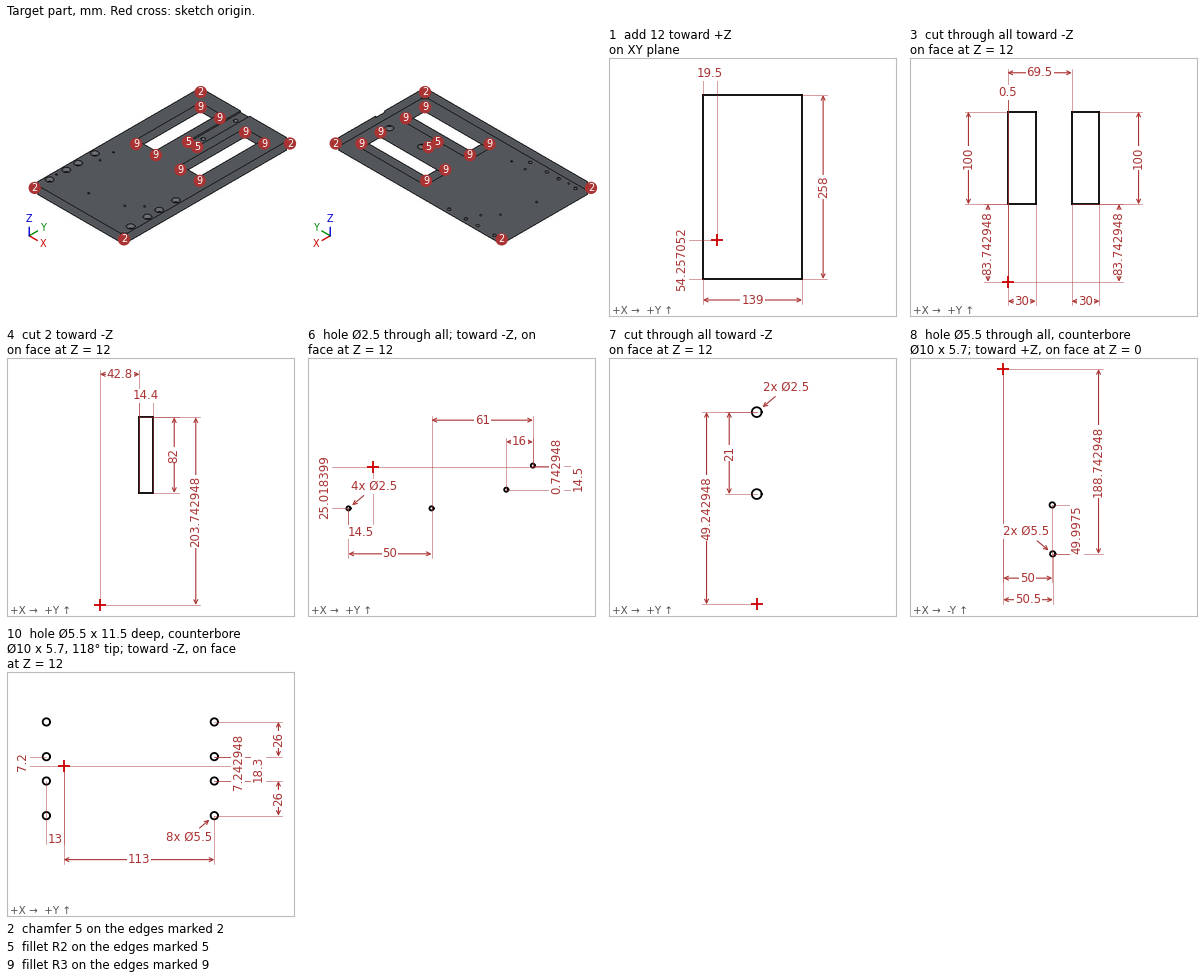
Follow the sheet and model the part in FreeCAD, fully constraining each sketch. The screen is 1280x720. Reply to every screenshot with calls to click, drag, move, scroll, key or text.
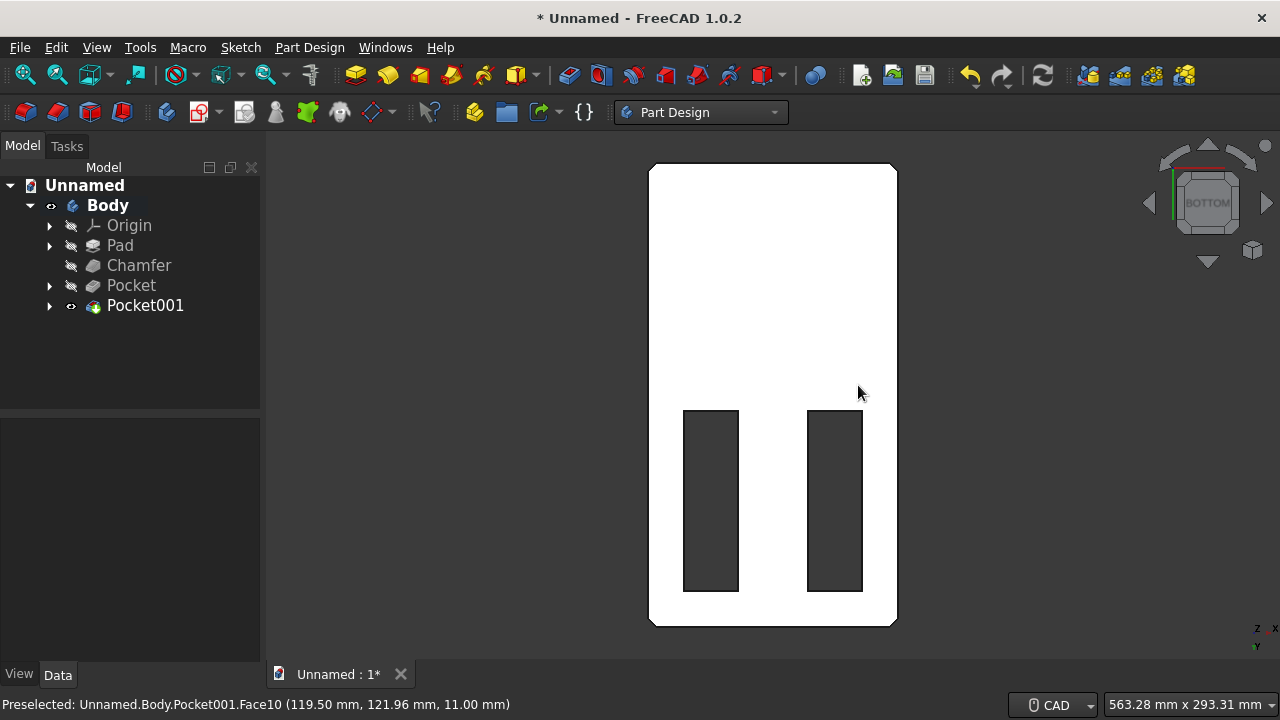
scroll(786, 479, up, 13)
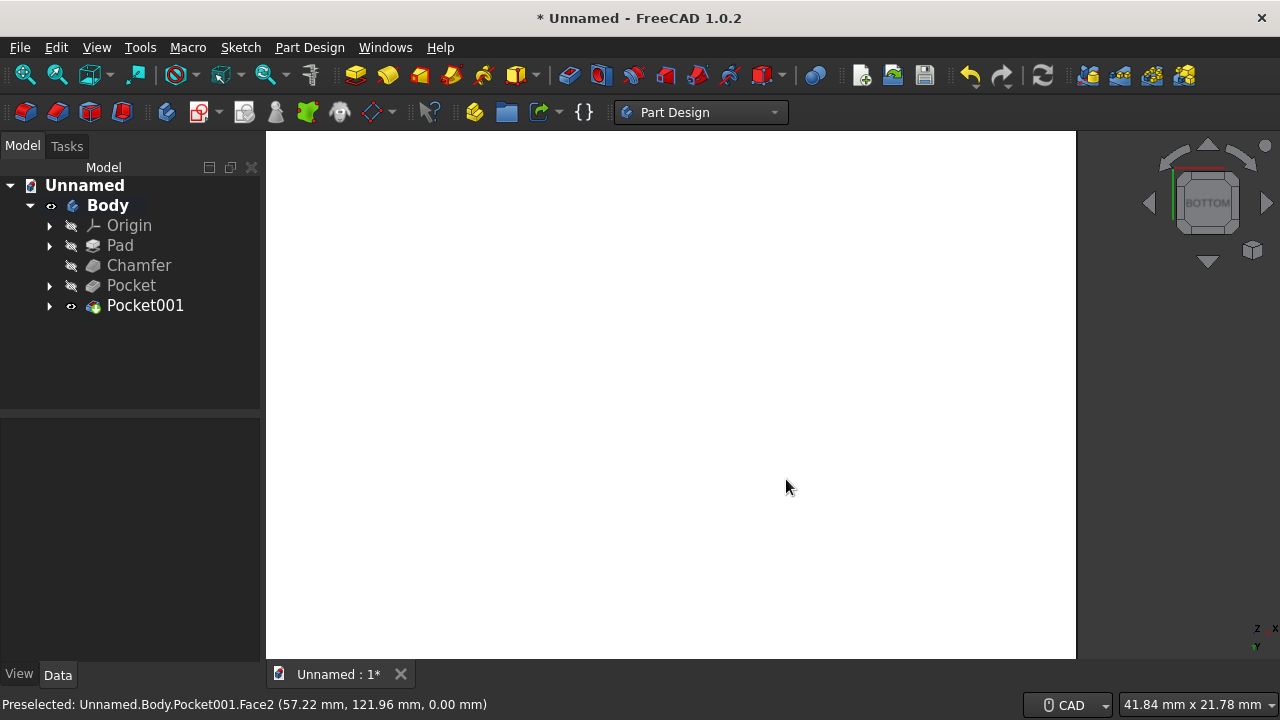
key(v)
key(f)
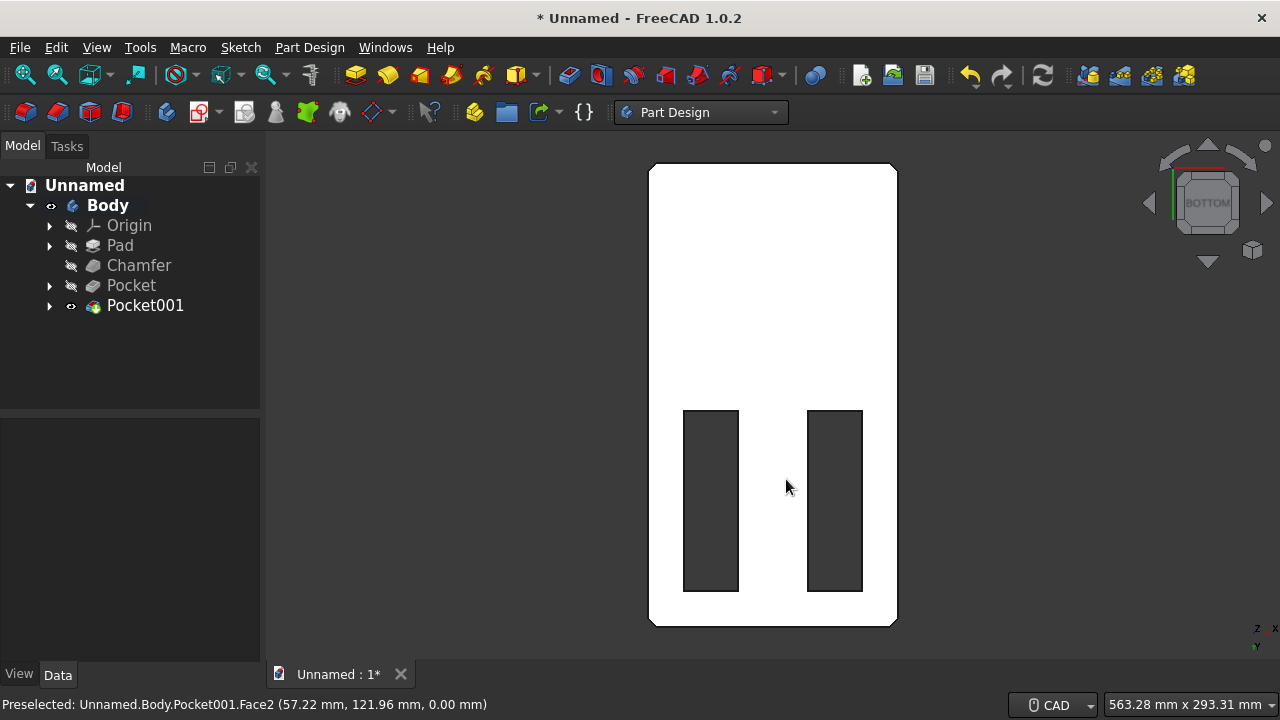
key(4)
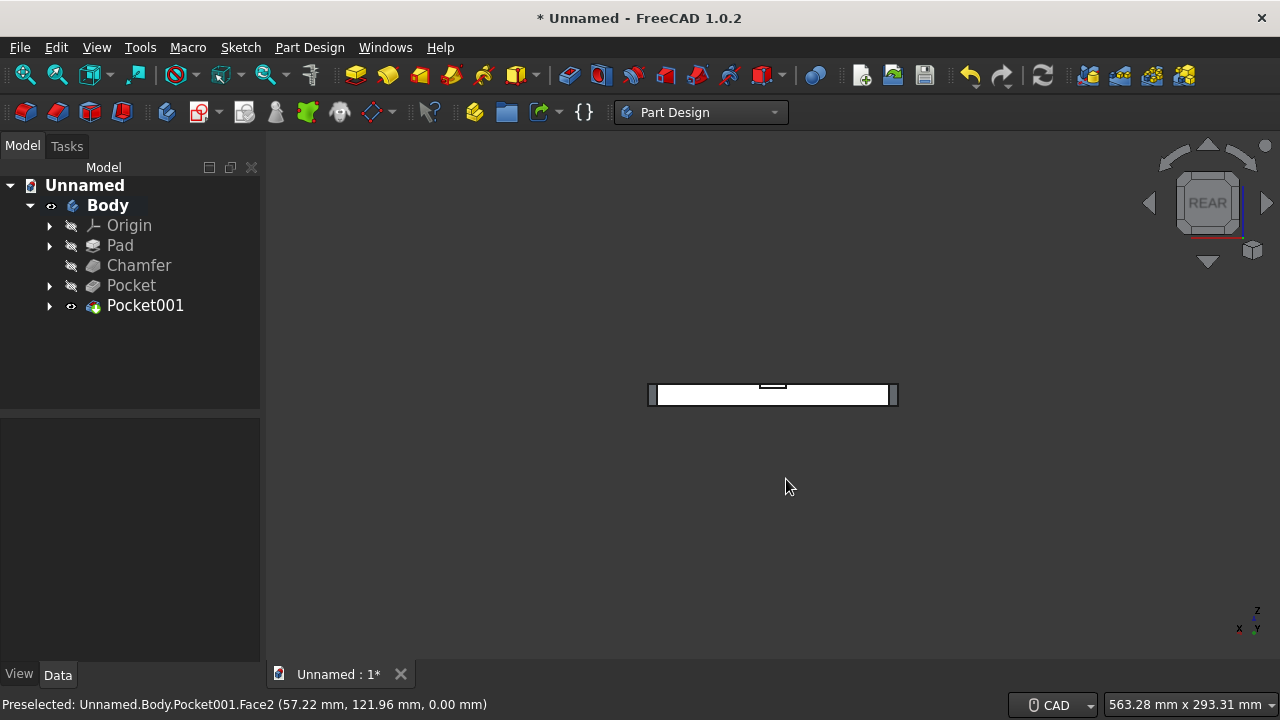
key(v)
key(f)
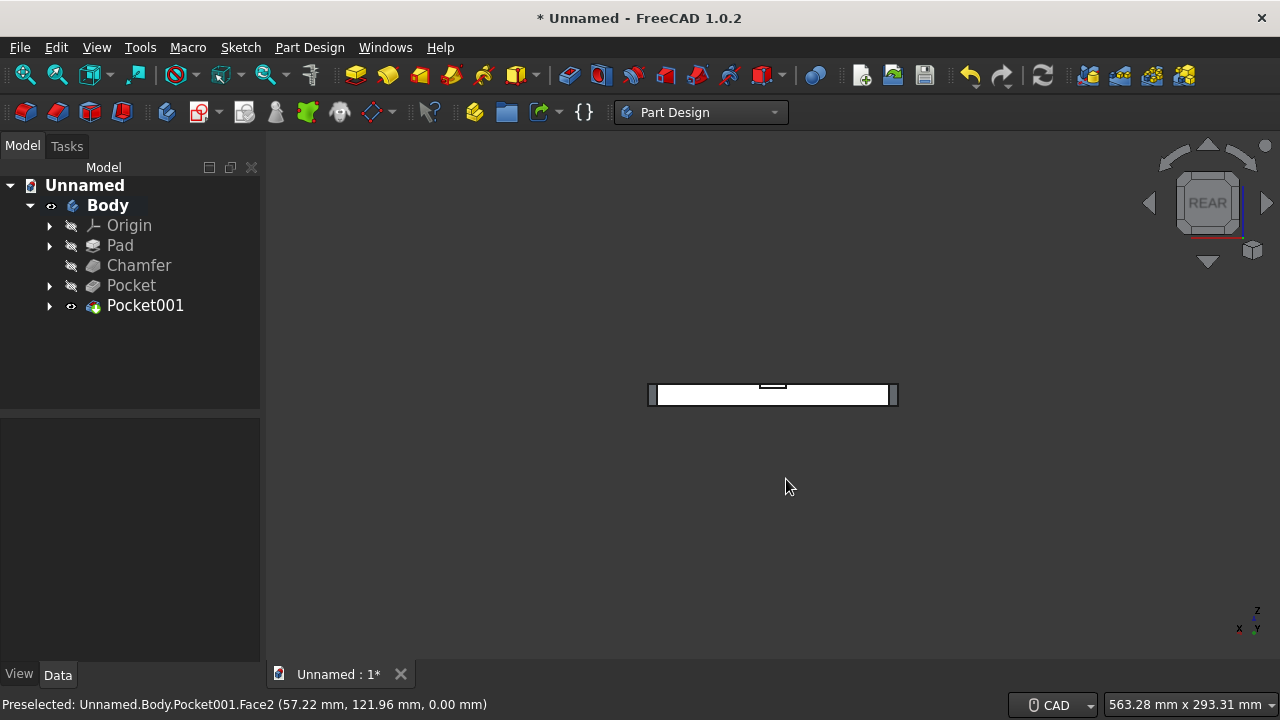
scroll(760, 385, up, 13)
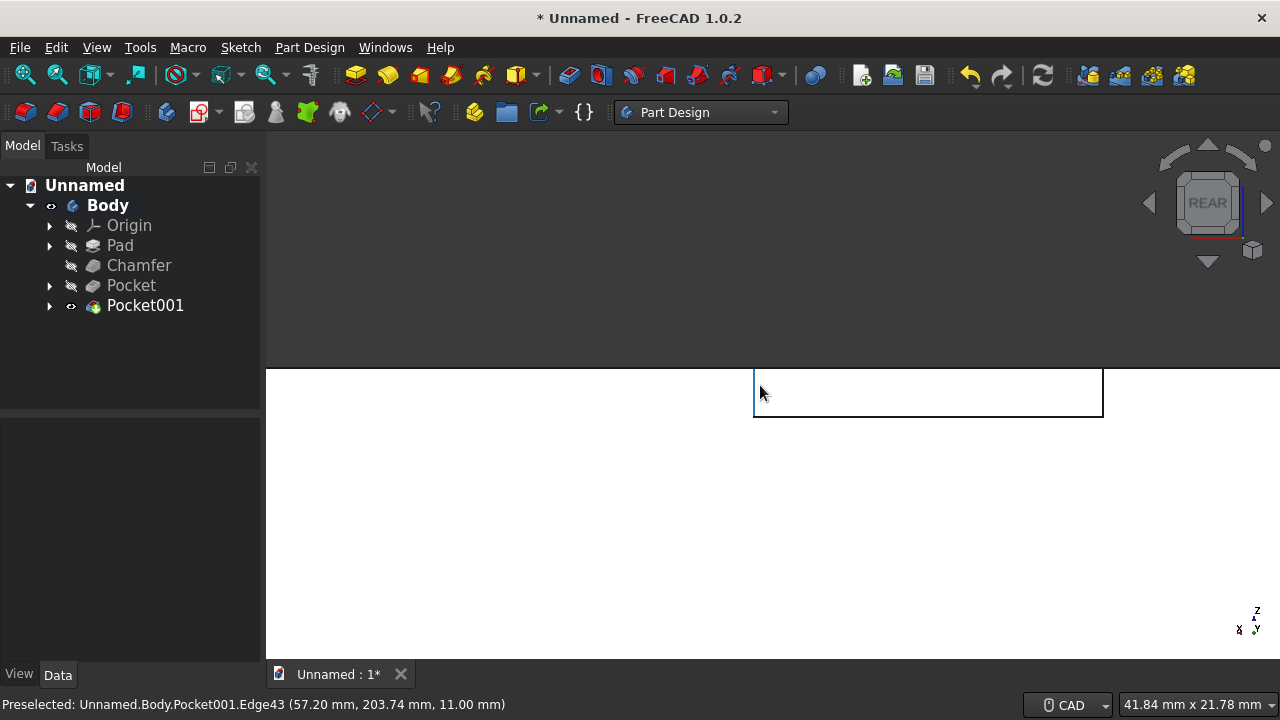
key(v)
key(f)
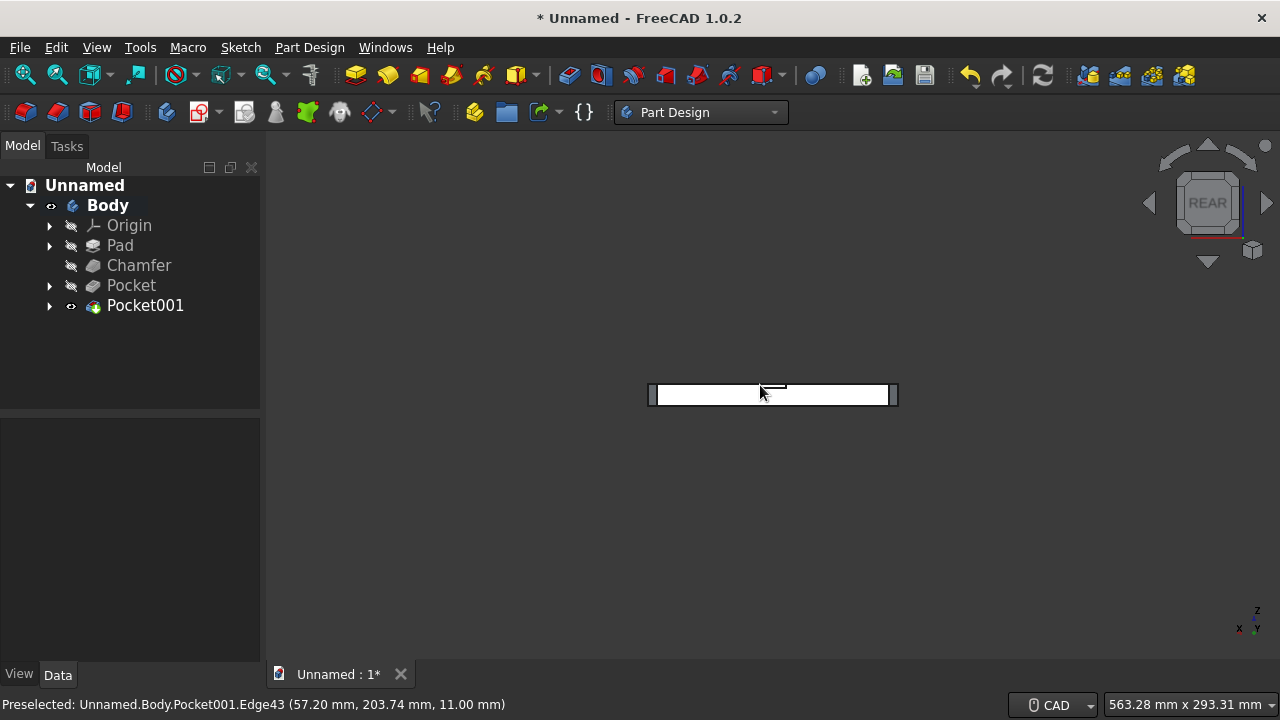
key(6)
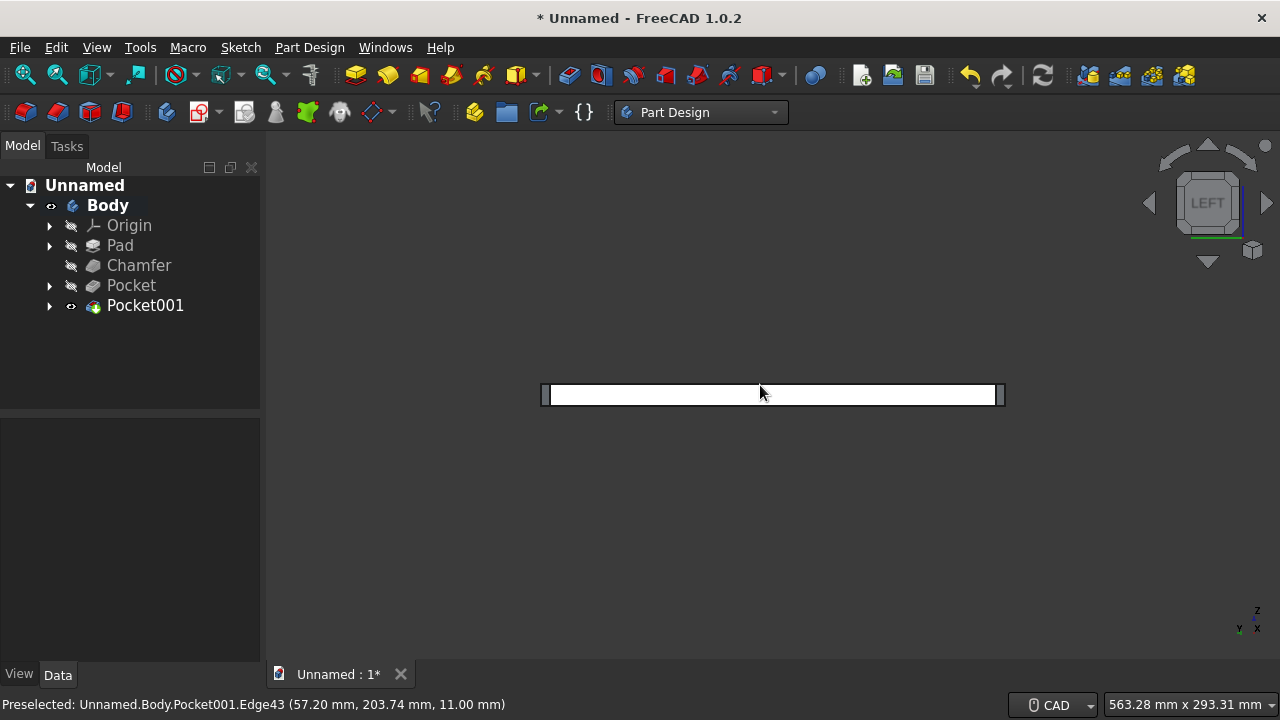
scroll(688, 385, up, 13)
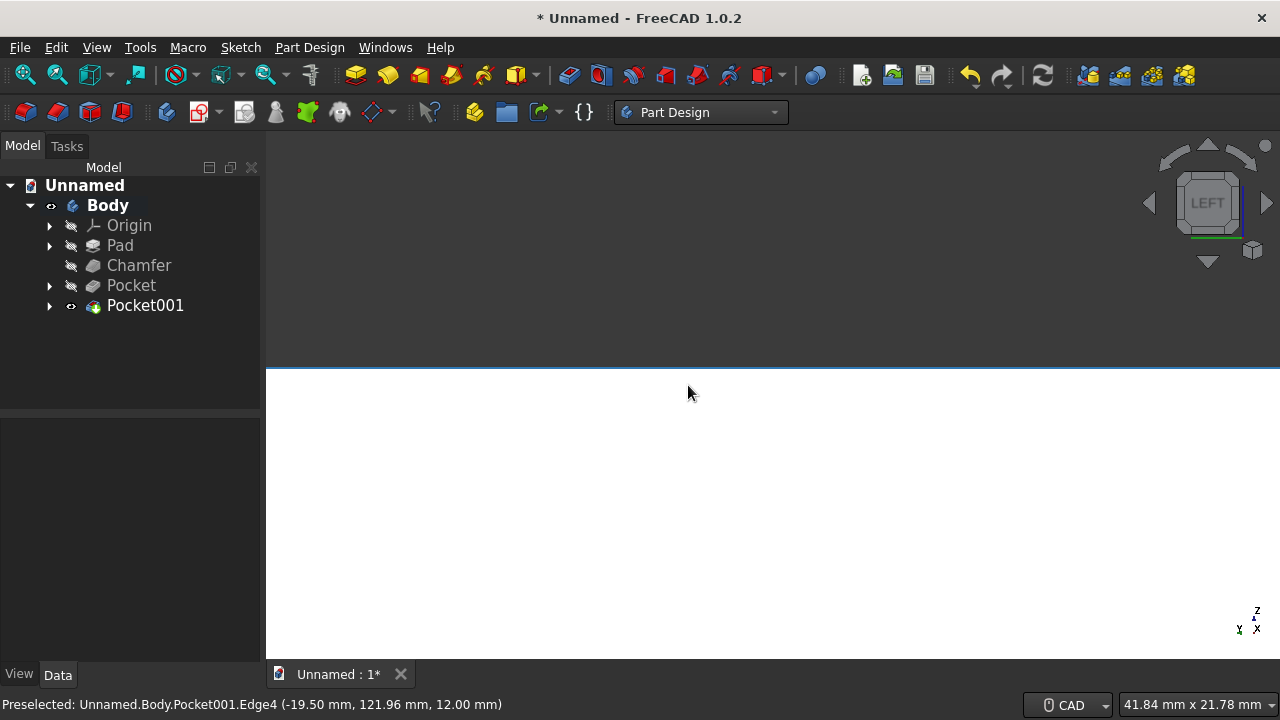
key(v)
key(f)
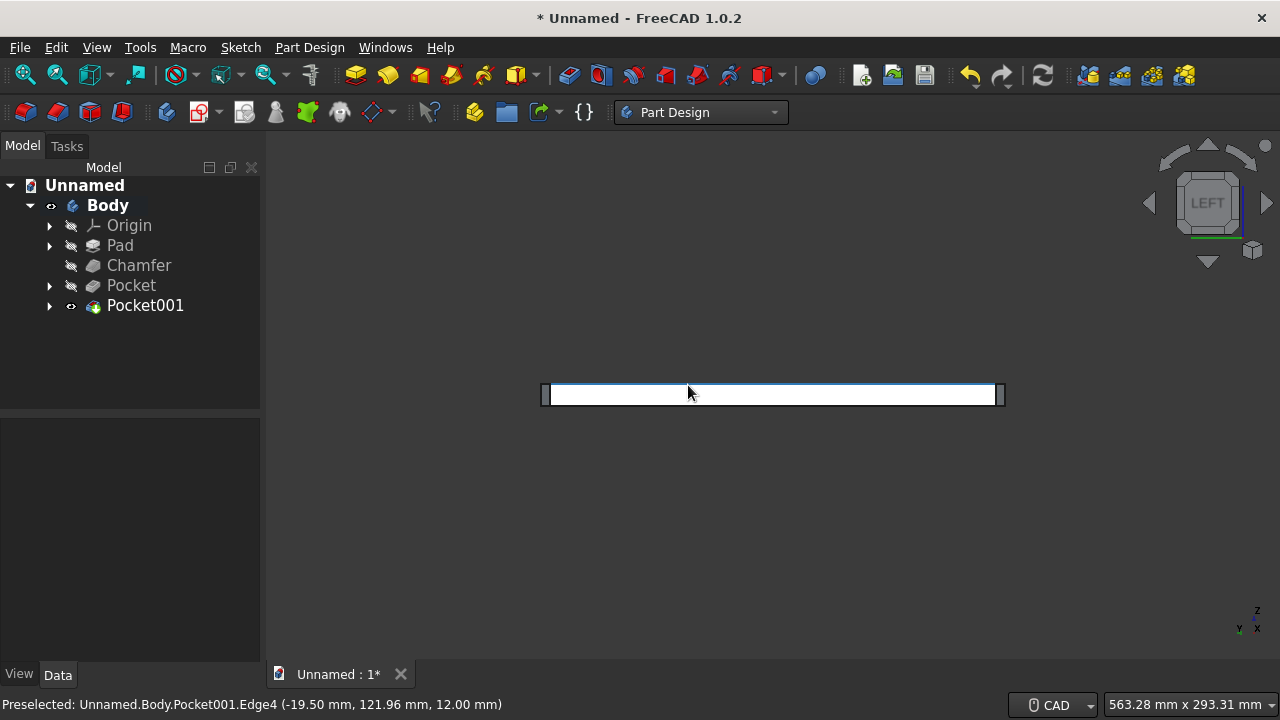
key(v)
key(3)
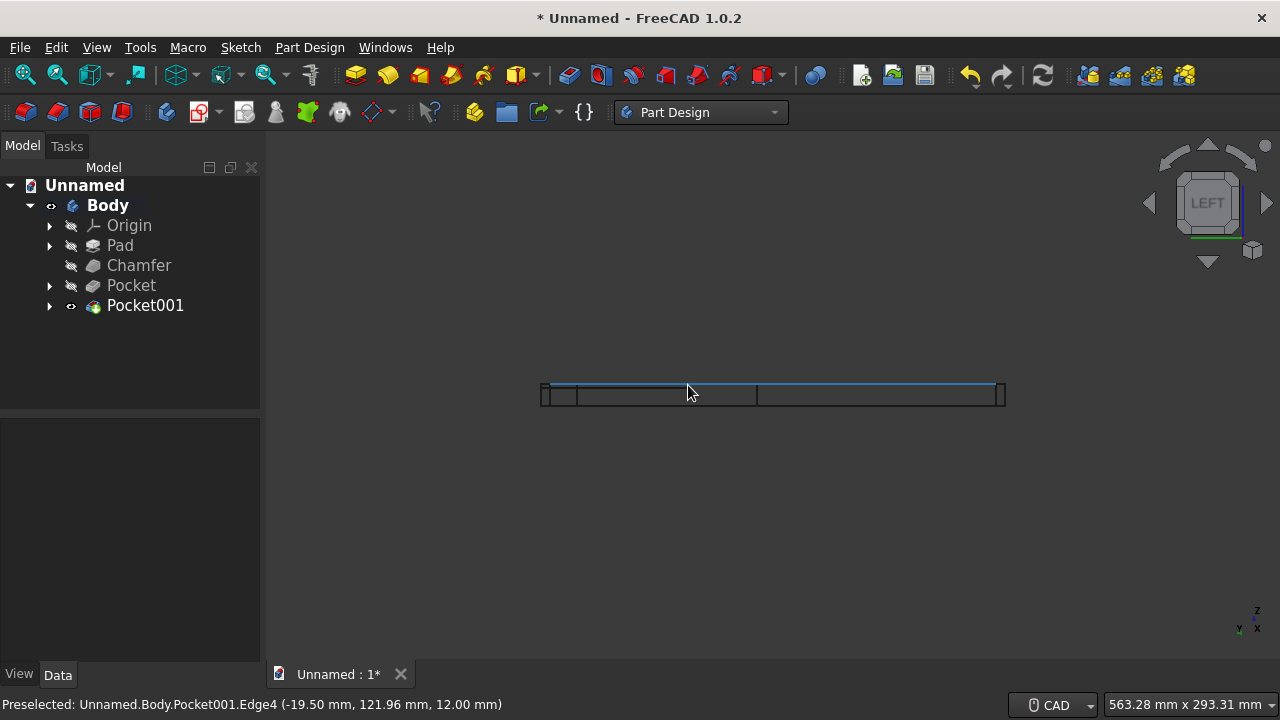
key(0)